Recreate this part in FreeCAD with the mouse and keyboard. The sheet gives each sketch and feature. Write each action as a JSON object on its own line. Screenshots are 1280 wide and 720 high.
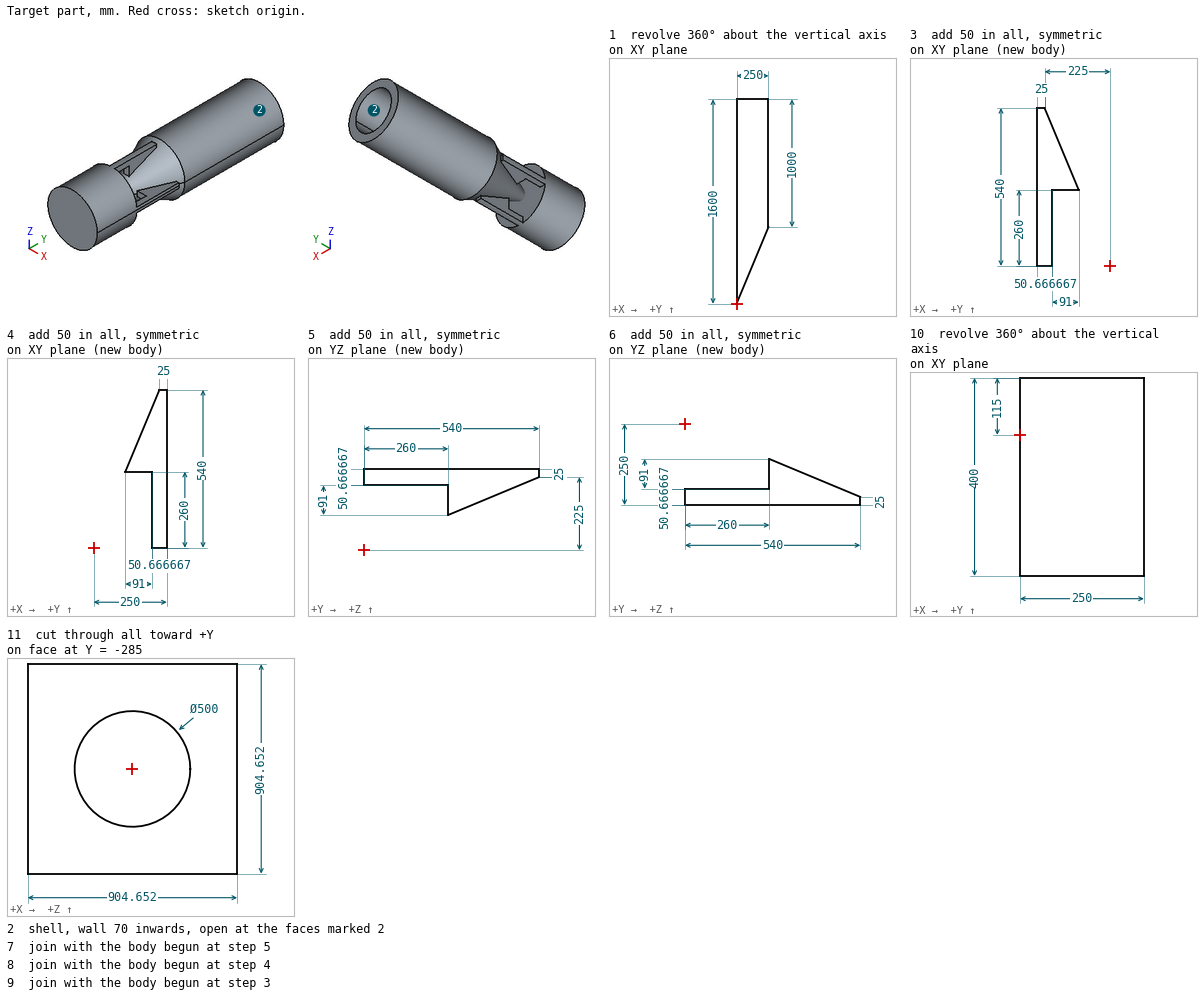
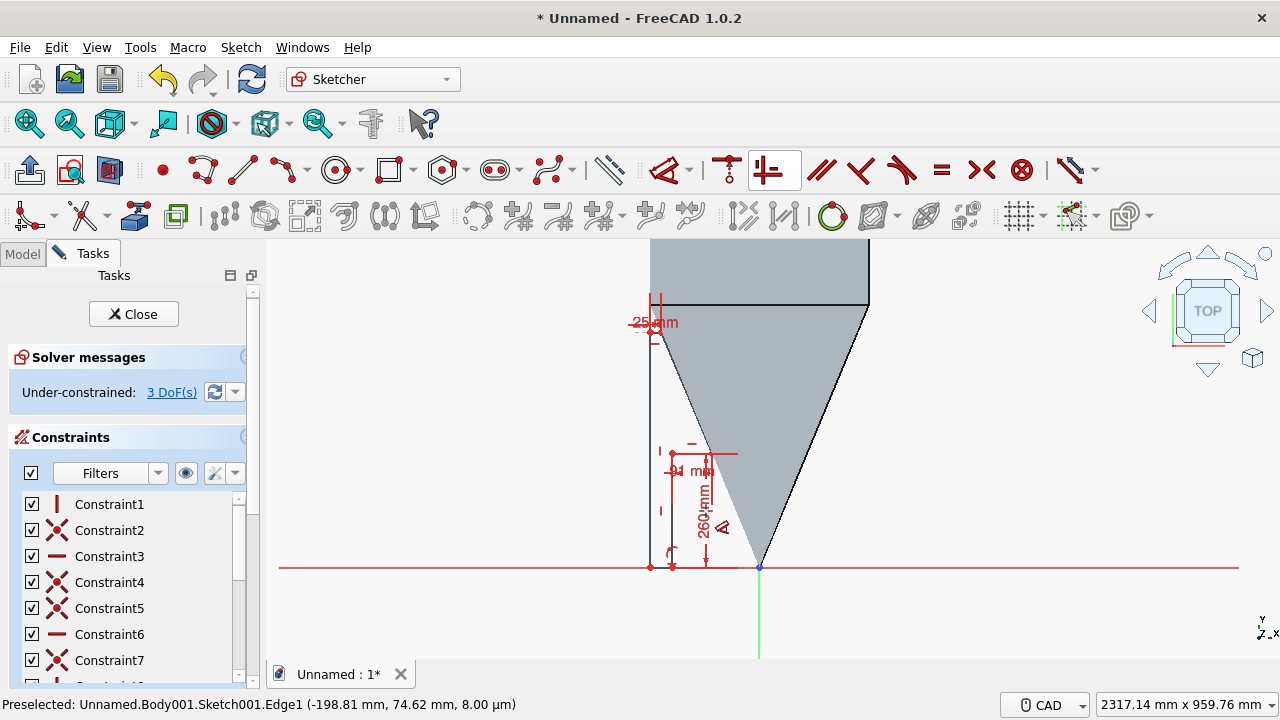
{"action": "left_click", "coordinate": [650, 403]}
{"action": "left_click", "coordinate": [616, 450]}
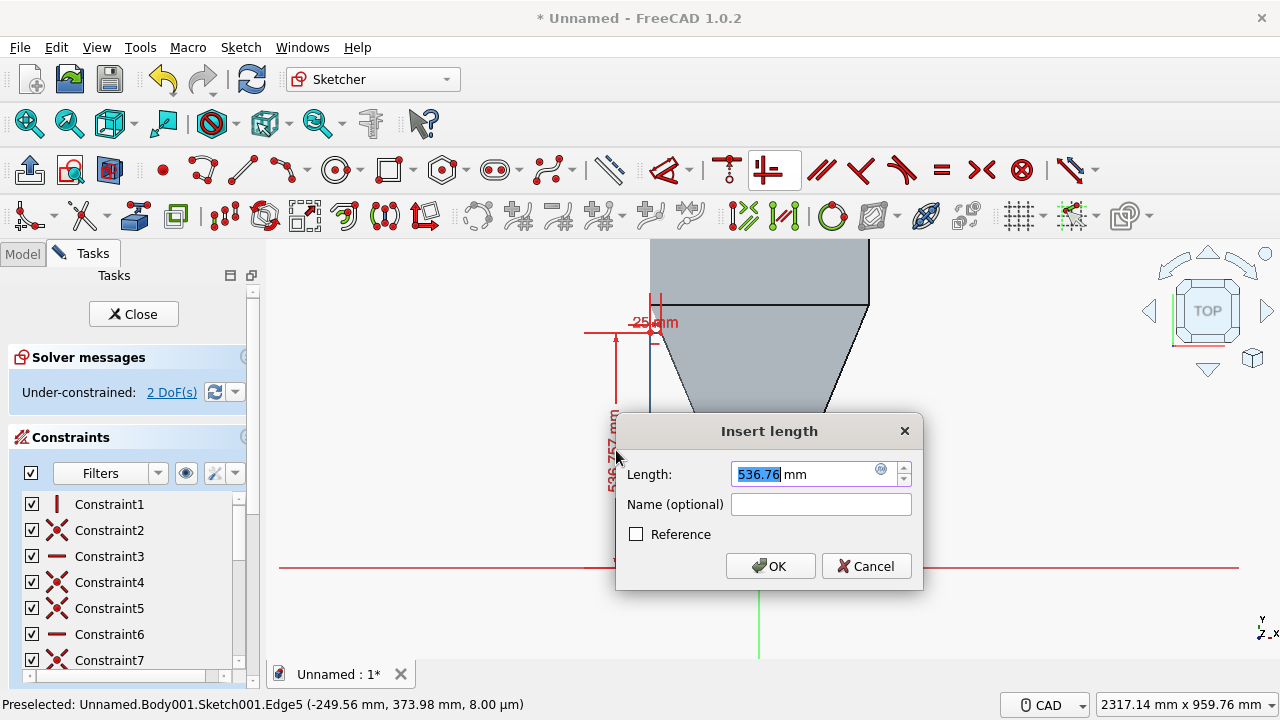
{"action": "type", "text": "540"}
{"action": "key", "text": "Return"}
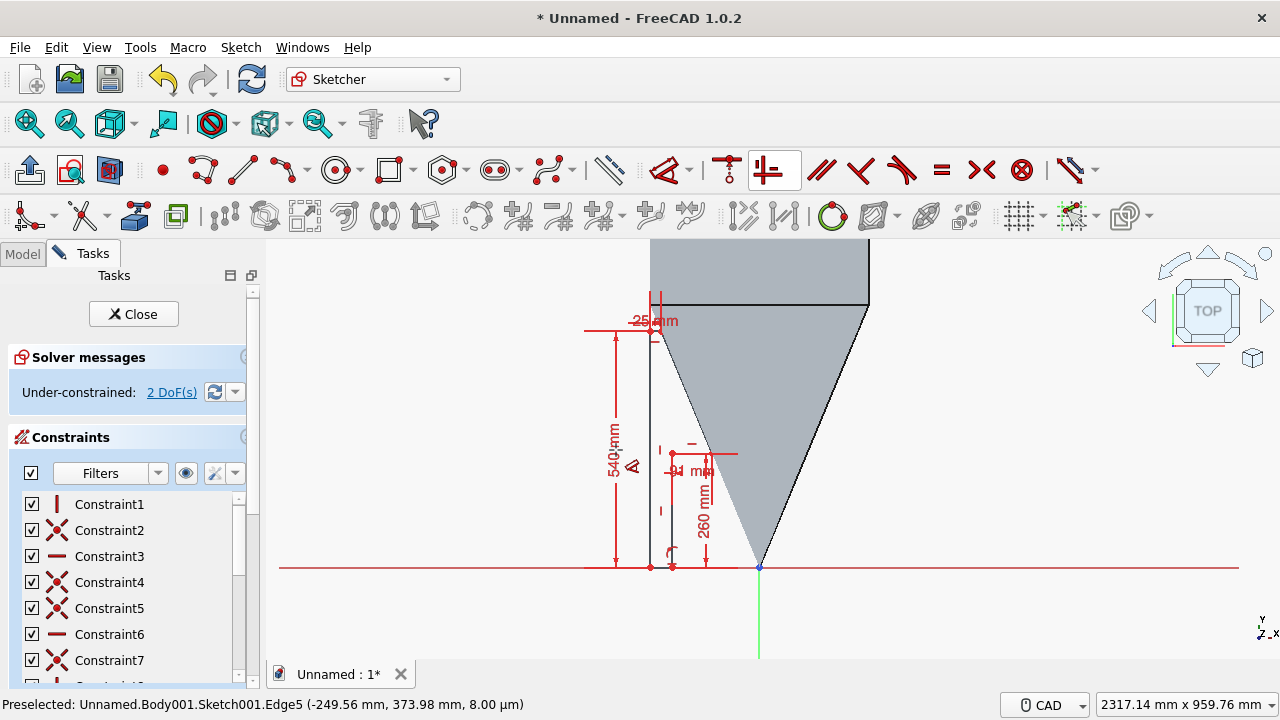
{"action": "left_click", "coordinate": [661, 331]}
{"action": "left_click", "coordinate": [710, 602]}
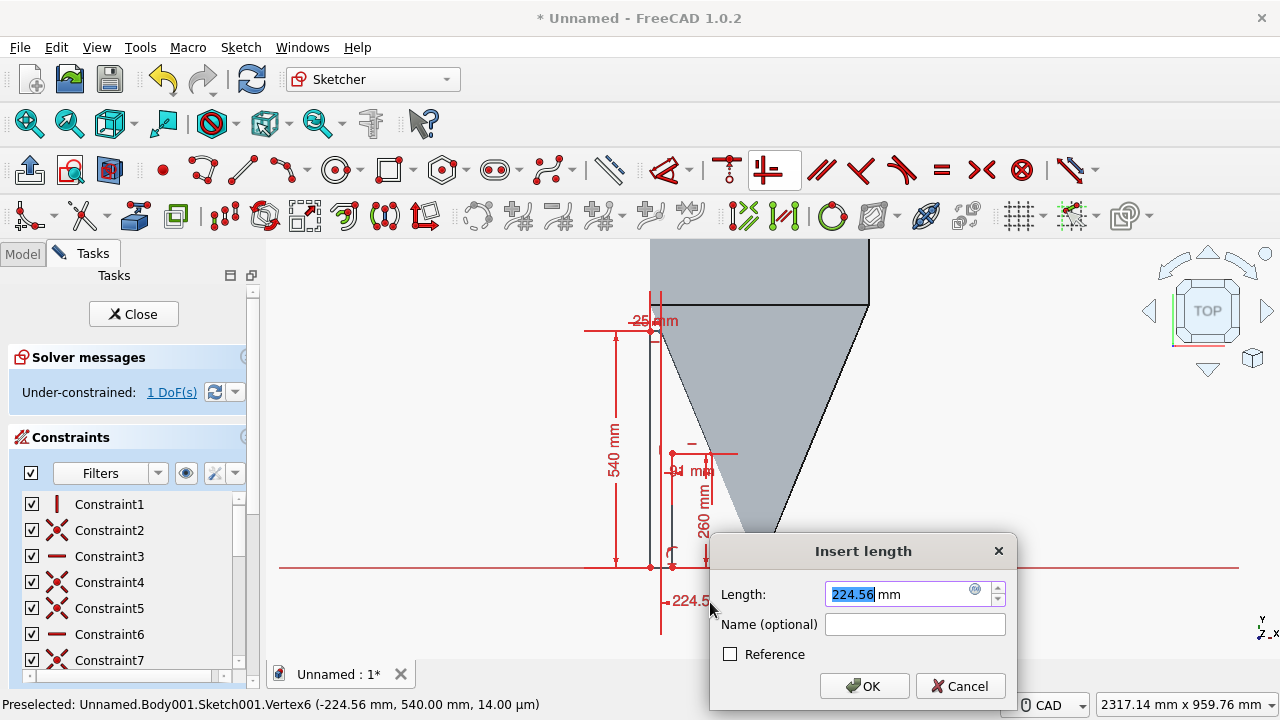
{"action": "type", "text": "225"}
{"action": "key", "text": "Return"}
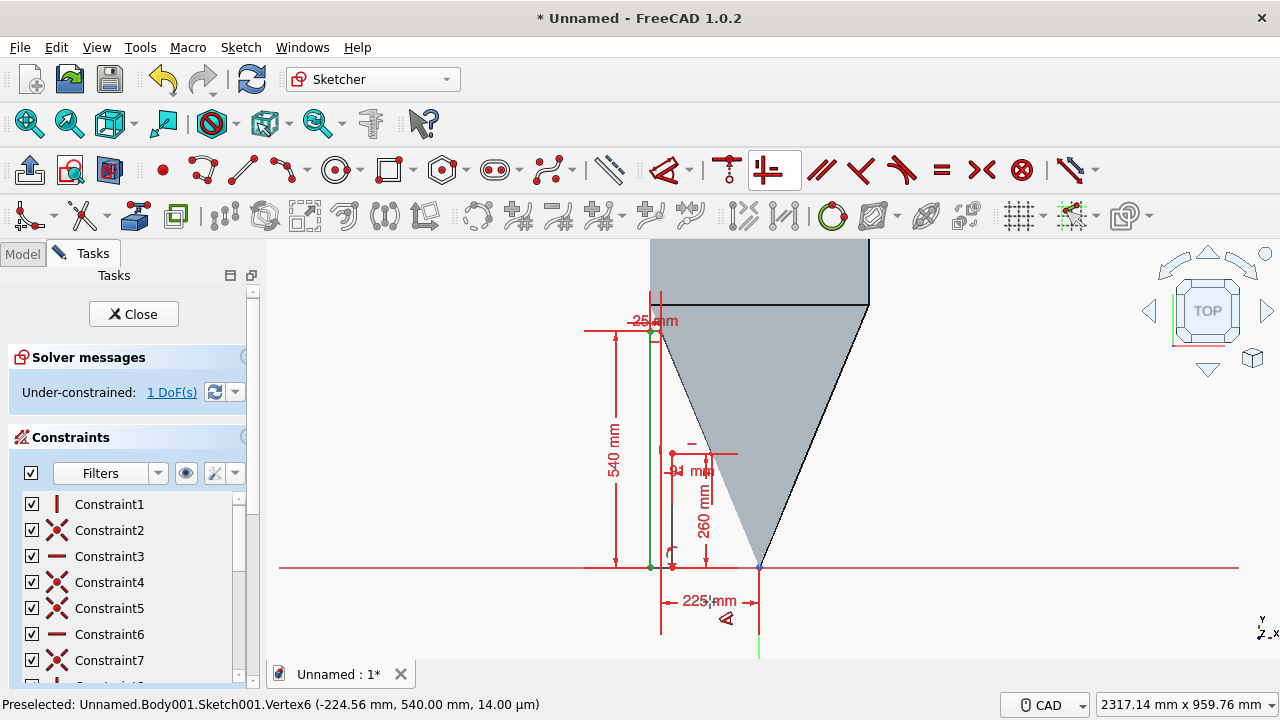
{"action": "scroll", "coordinate": [661, 568], "scroll_direction": "up", "scroll_amount": 3}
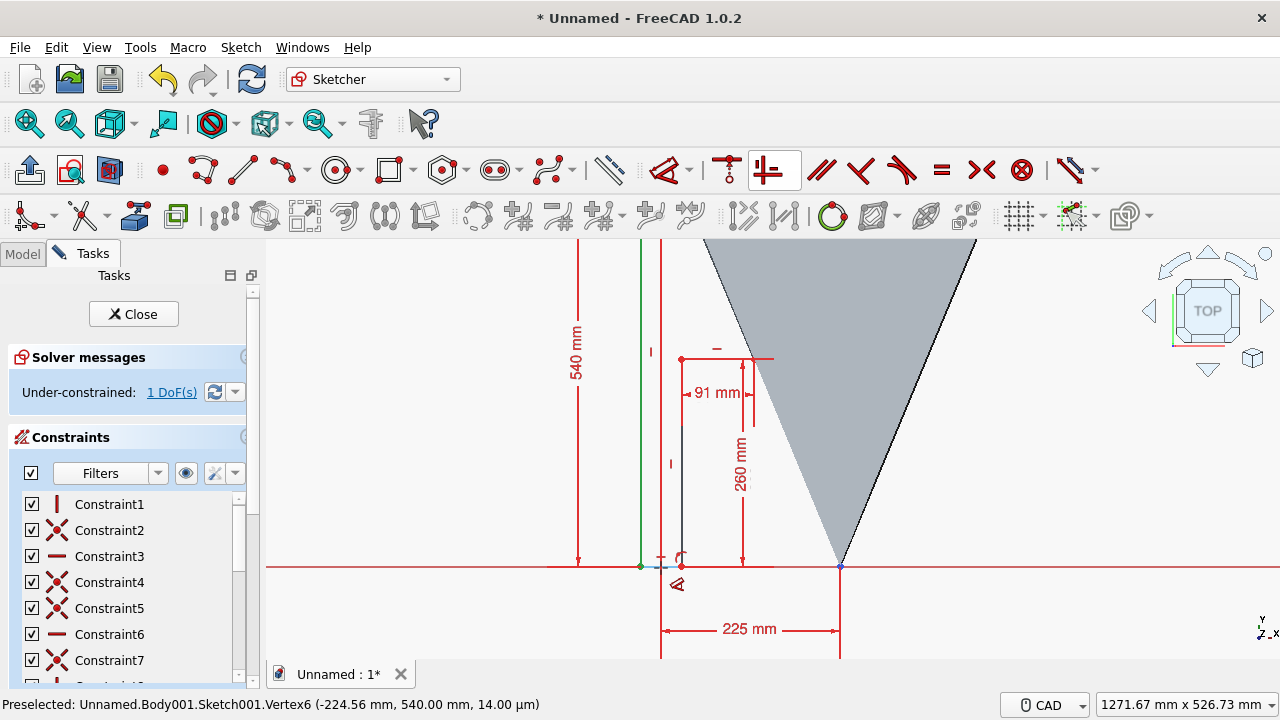
{"action": "left_click", "coordinate": [661, 567]}
{"action": "left_click", "coordinate": [661, 601]}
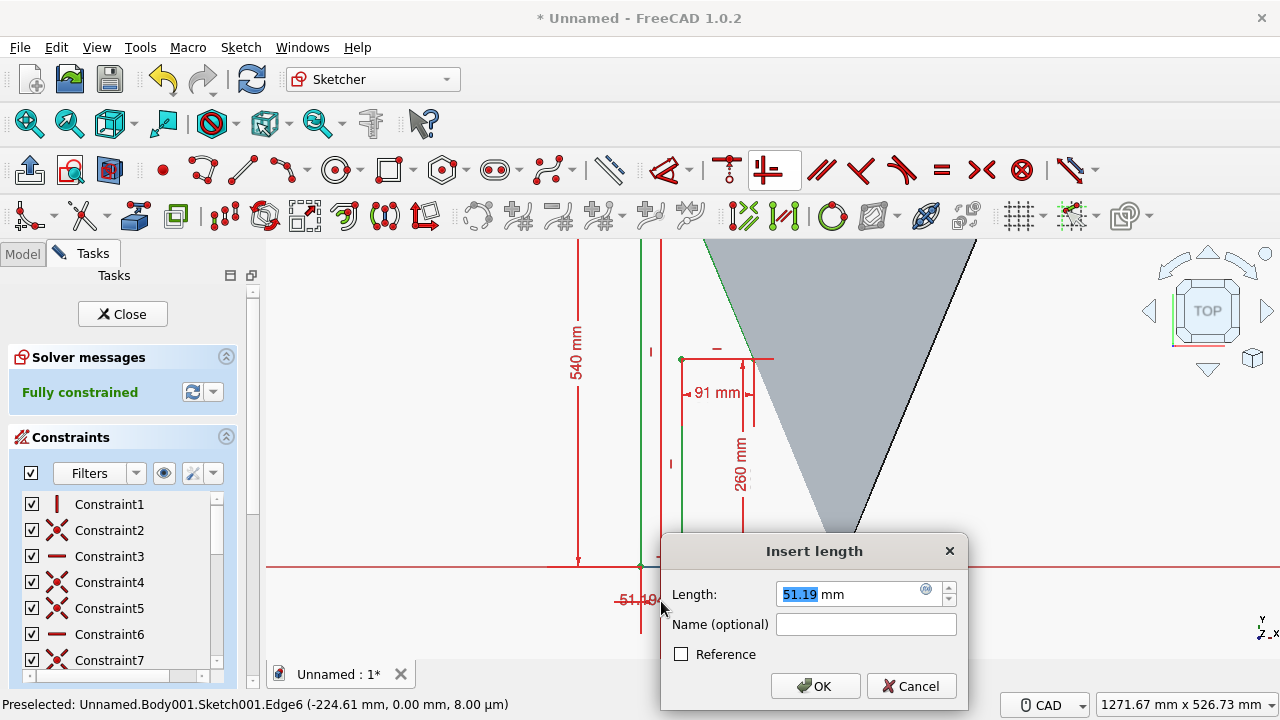
{"action": "type", "text": "50.666667"}
{"action": "key", "text": "Return"}
{"action": "key", "text": "Escape"}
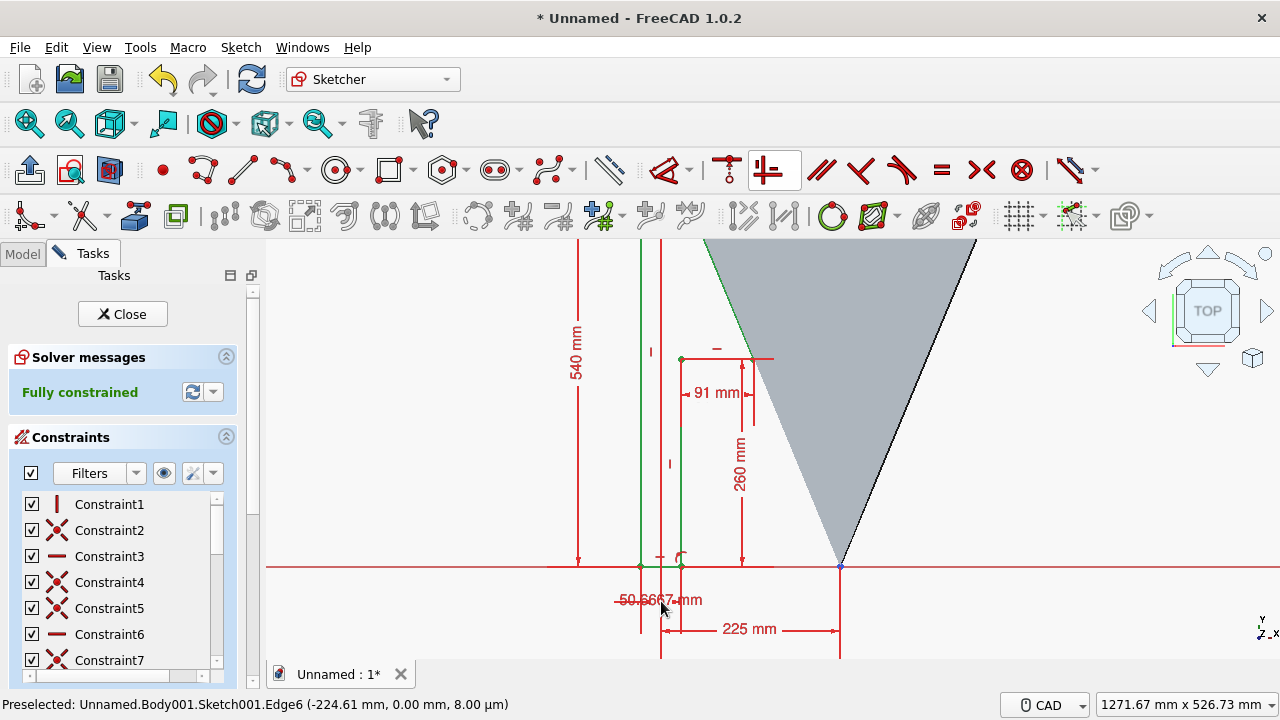
{"action": "left_click", "coordinate": [123, 314]}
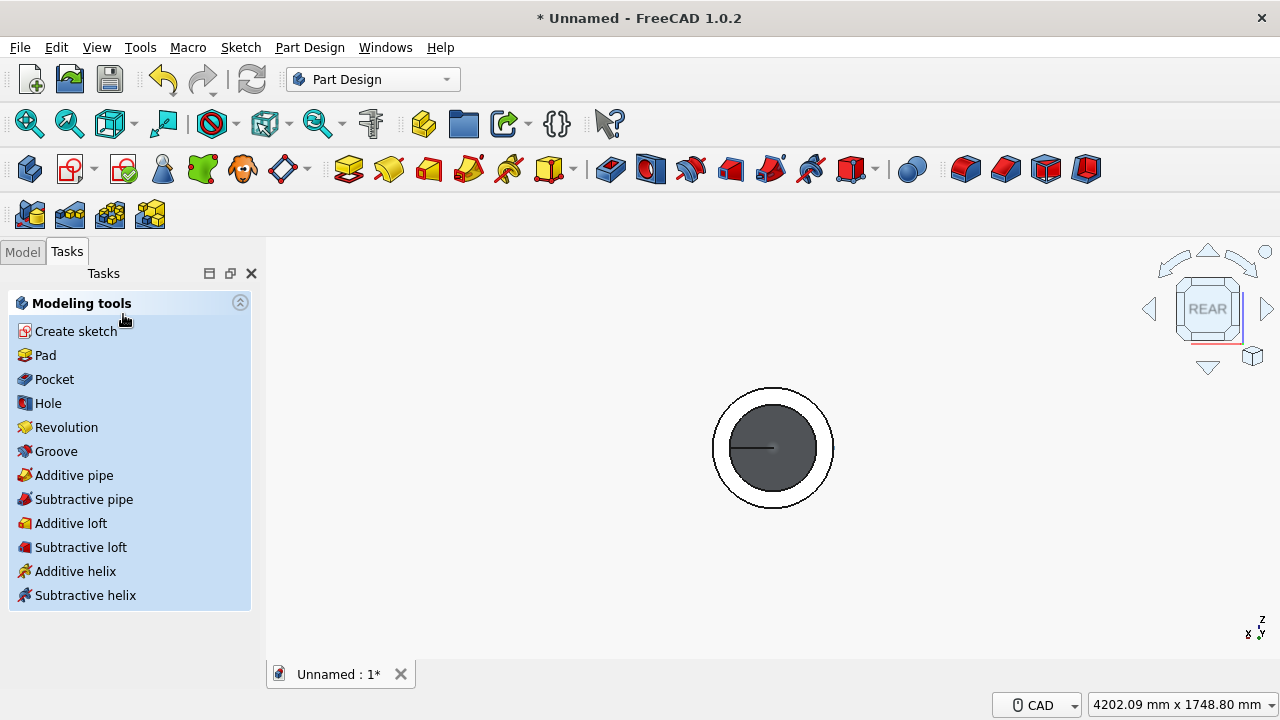
{"action": "left_click", "coordinate": [350, 170]}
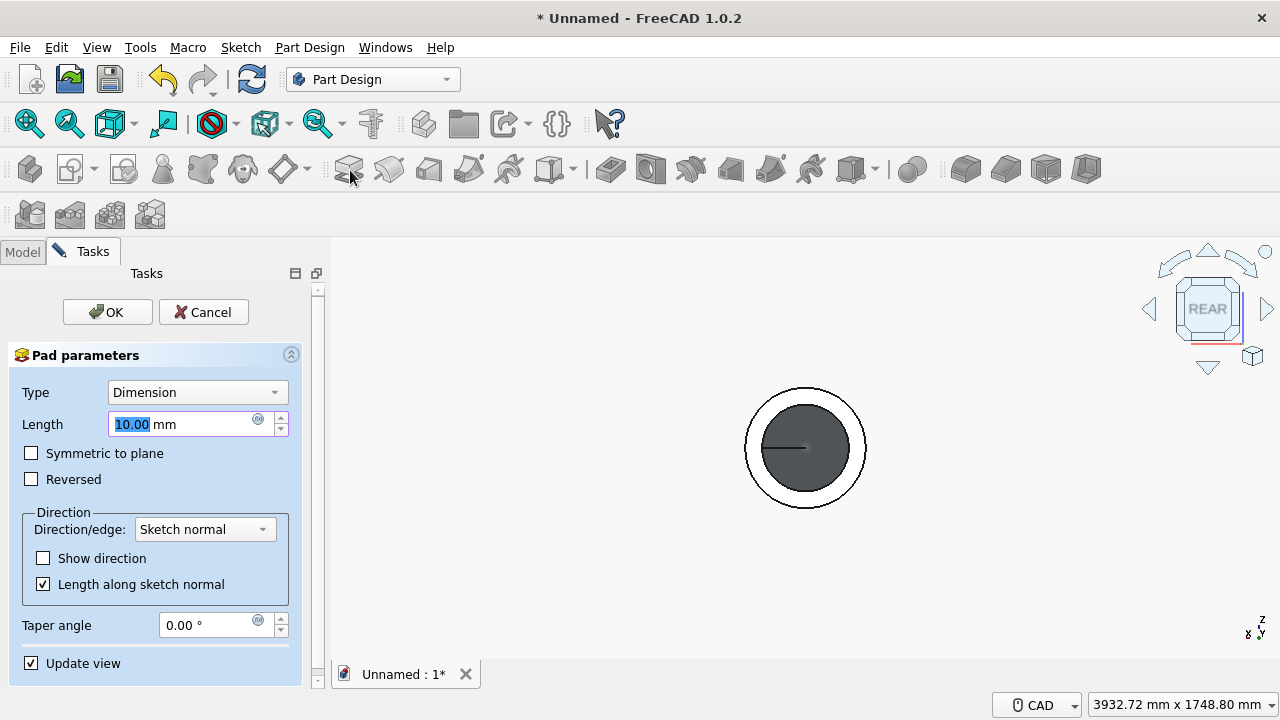
{"action": "type", "text": "50"}
{"action": "key", "text": "Tab"}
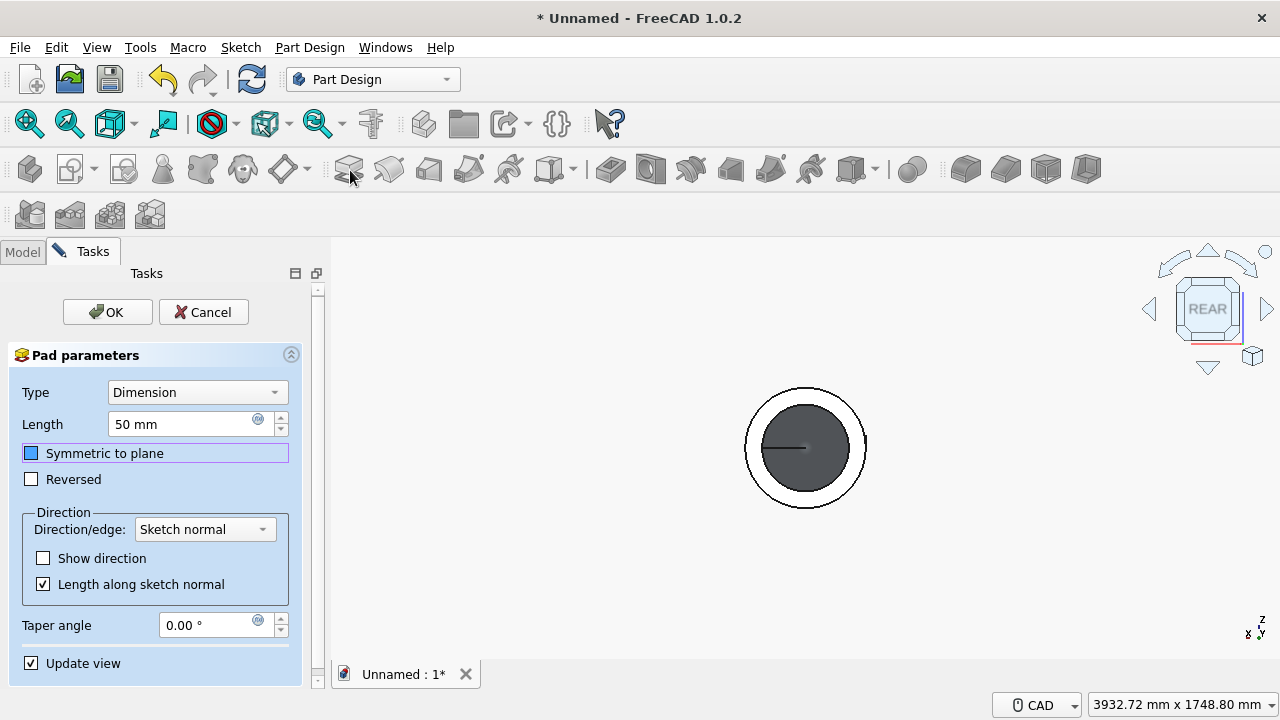
{"action": "left_click", "coordinate": [30, 453]}